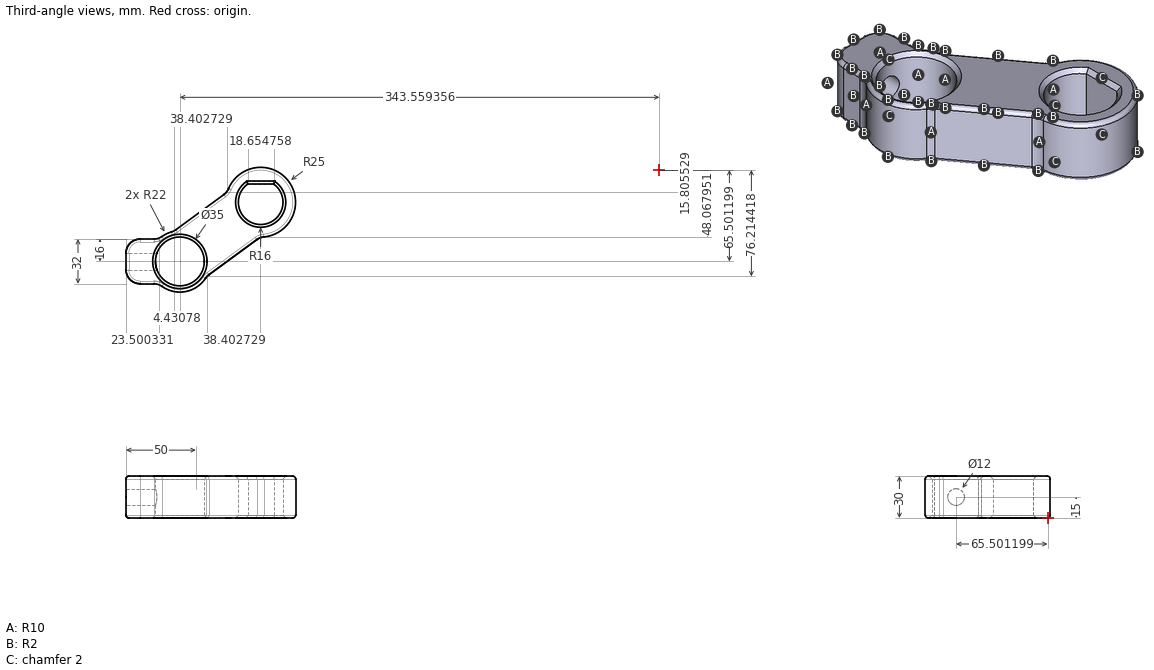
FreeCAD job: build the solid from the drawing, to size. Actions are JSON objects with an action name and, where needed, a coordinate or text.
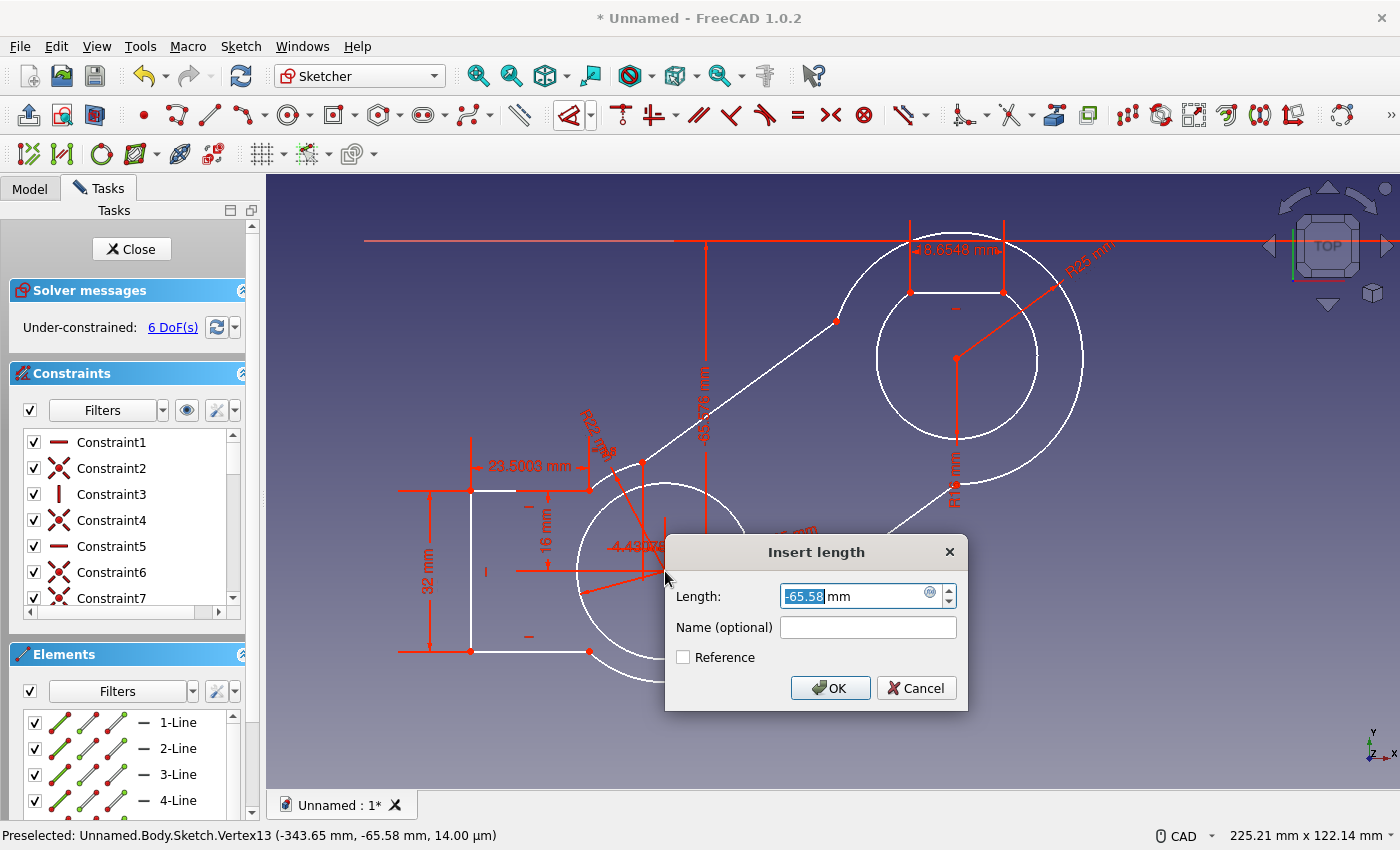
{"action": "type", "text": "-65.501199"}
{"action": "key", "text": "Return"}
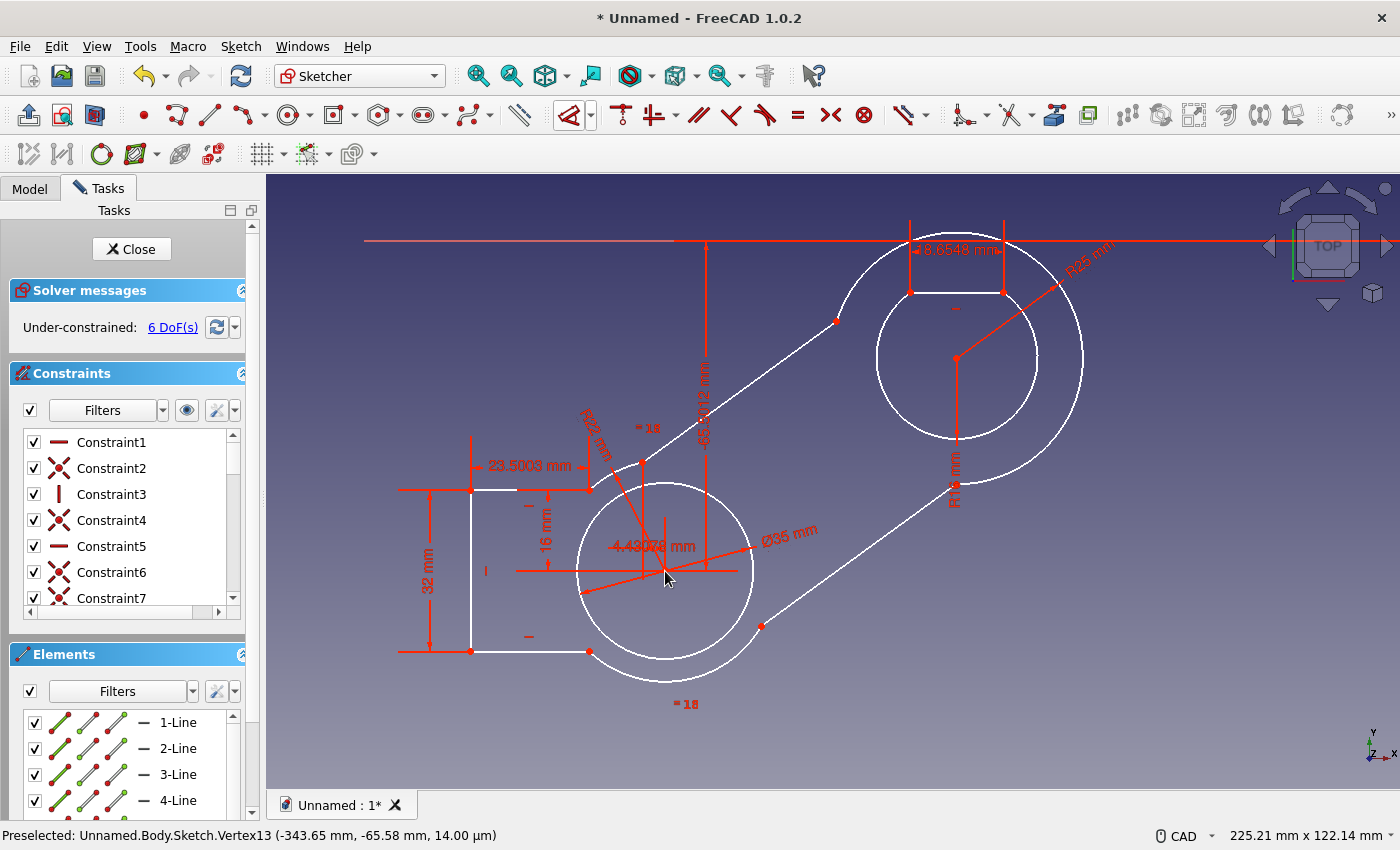
{"action": "left_click", "coordinate": [837, 321]}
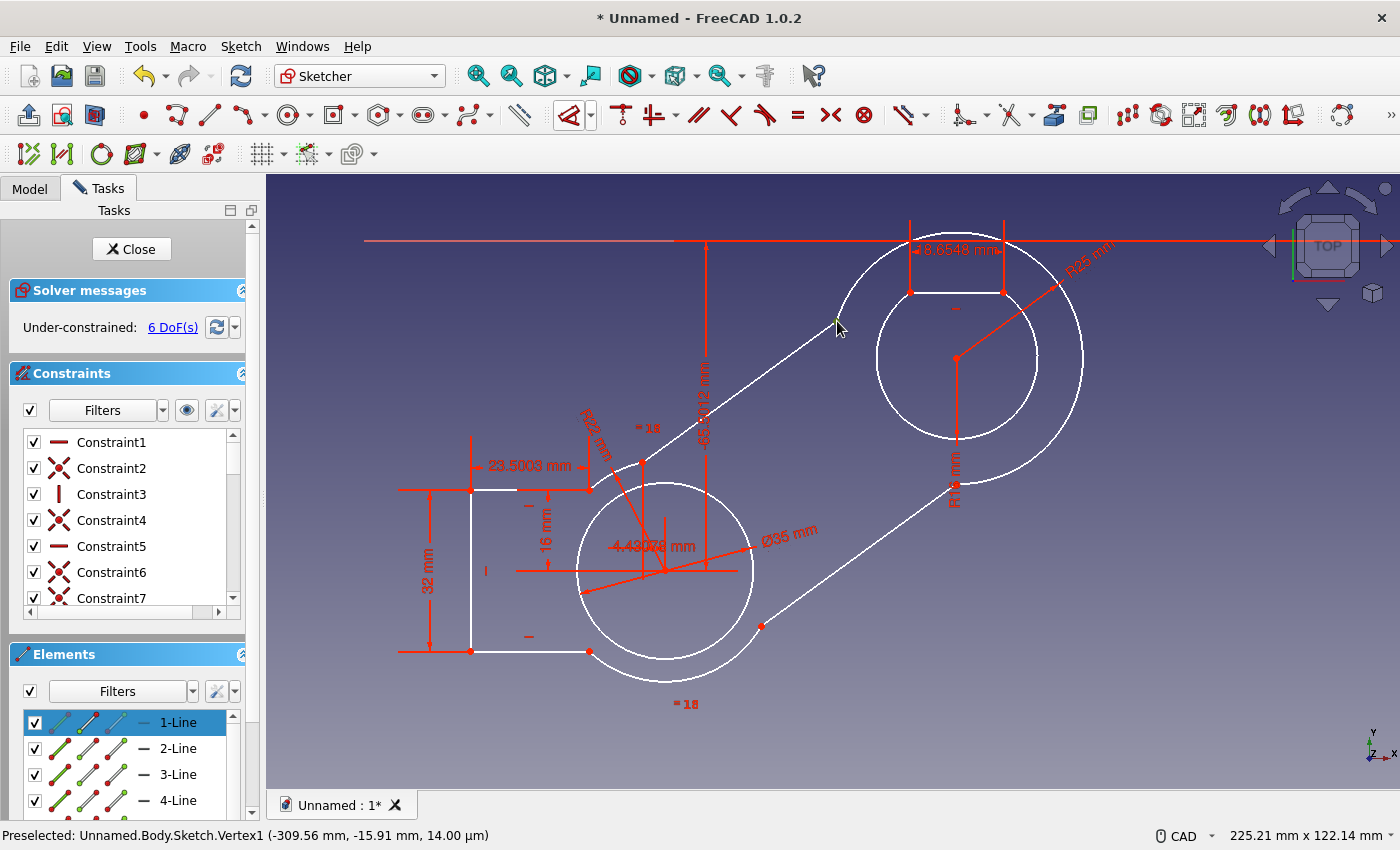
{"action": "key", "text": "i"}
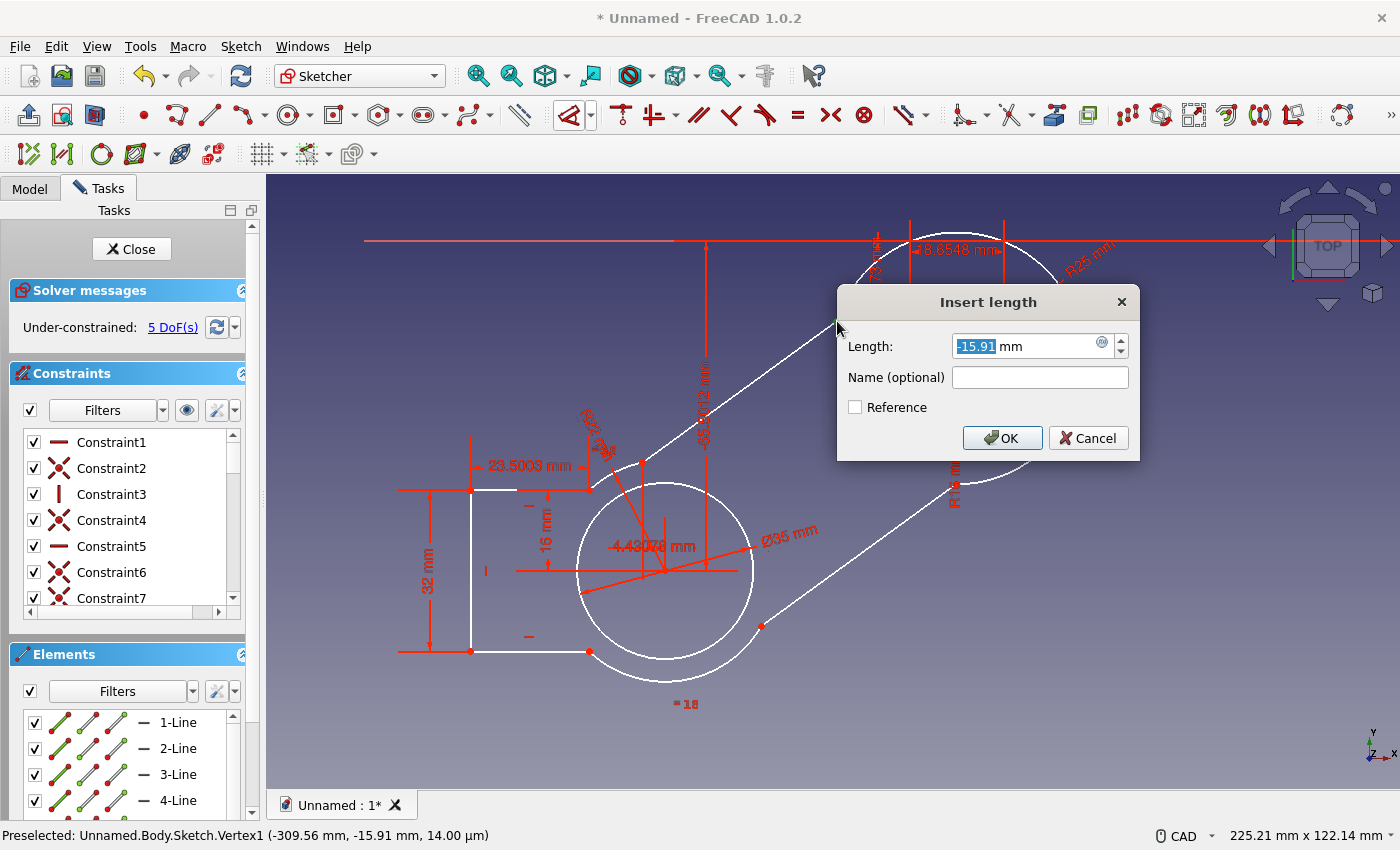
{"action": "type", "text": "-15.805529"}
{"action": "key", "text": "Return"}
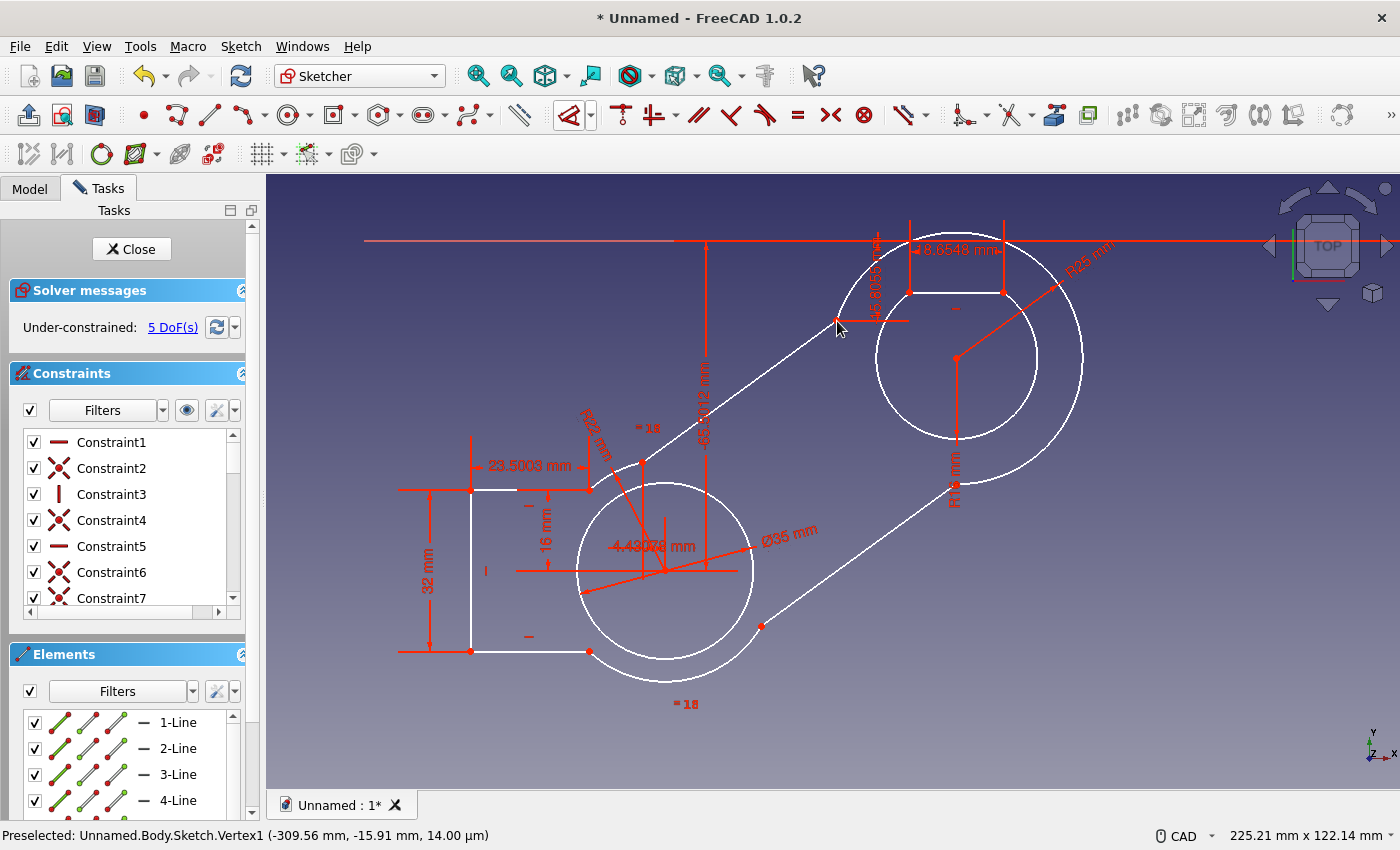
{"action": "left_click", "coordinate": [761, 626]}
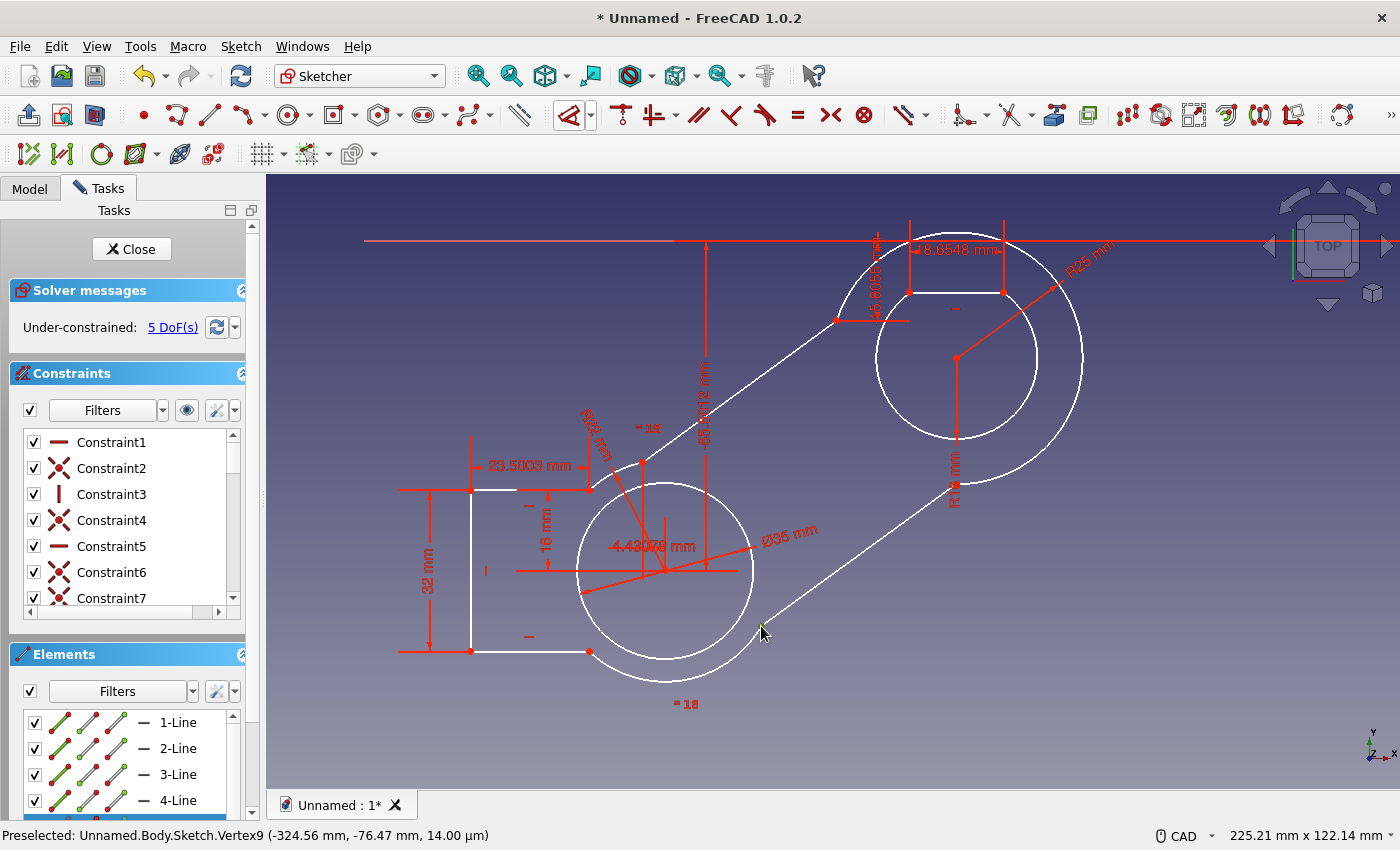
{"action": "left_click", "coordinate": [590, 116]}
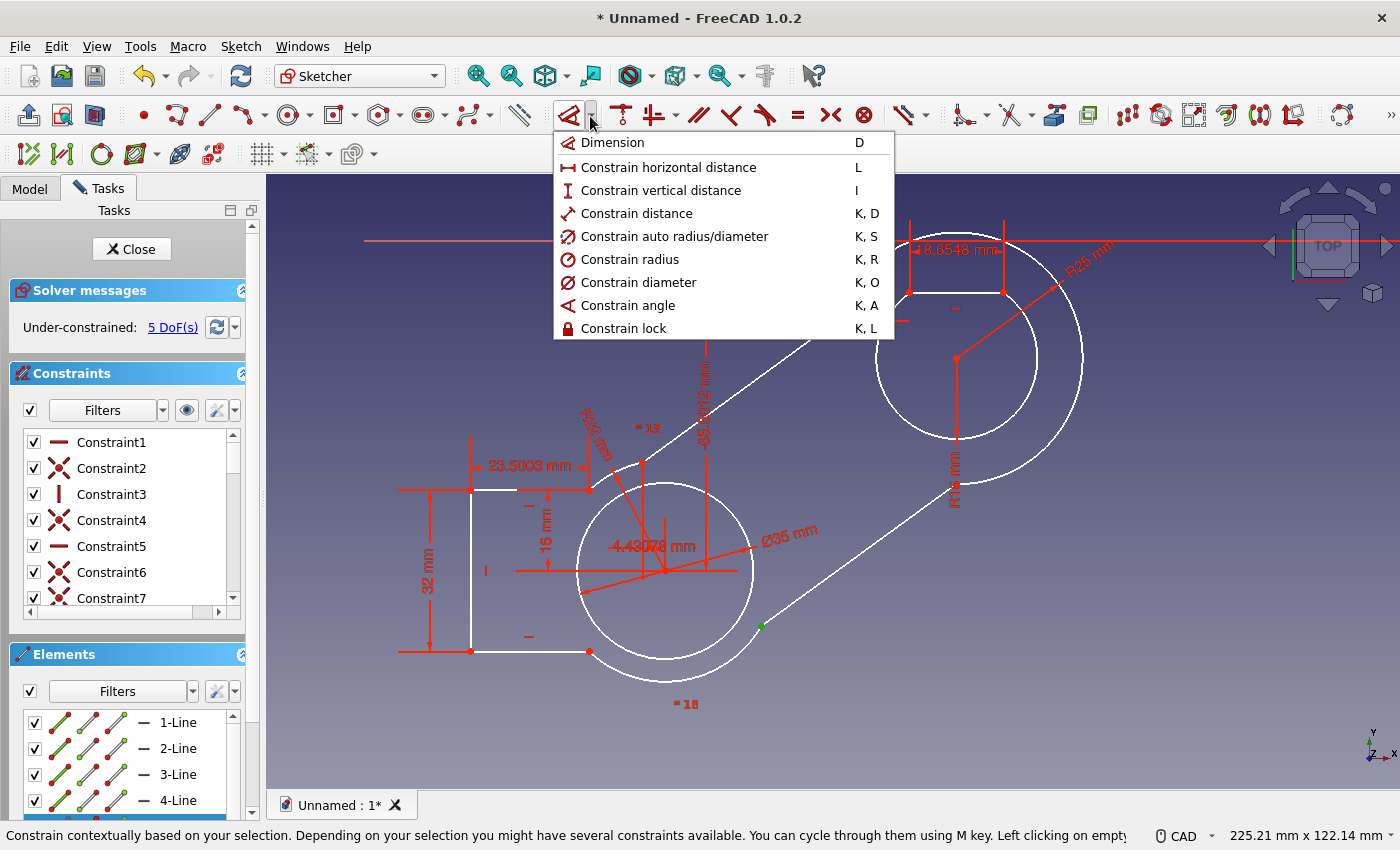
{"action": "left_click", "coordinate": [724, 190]}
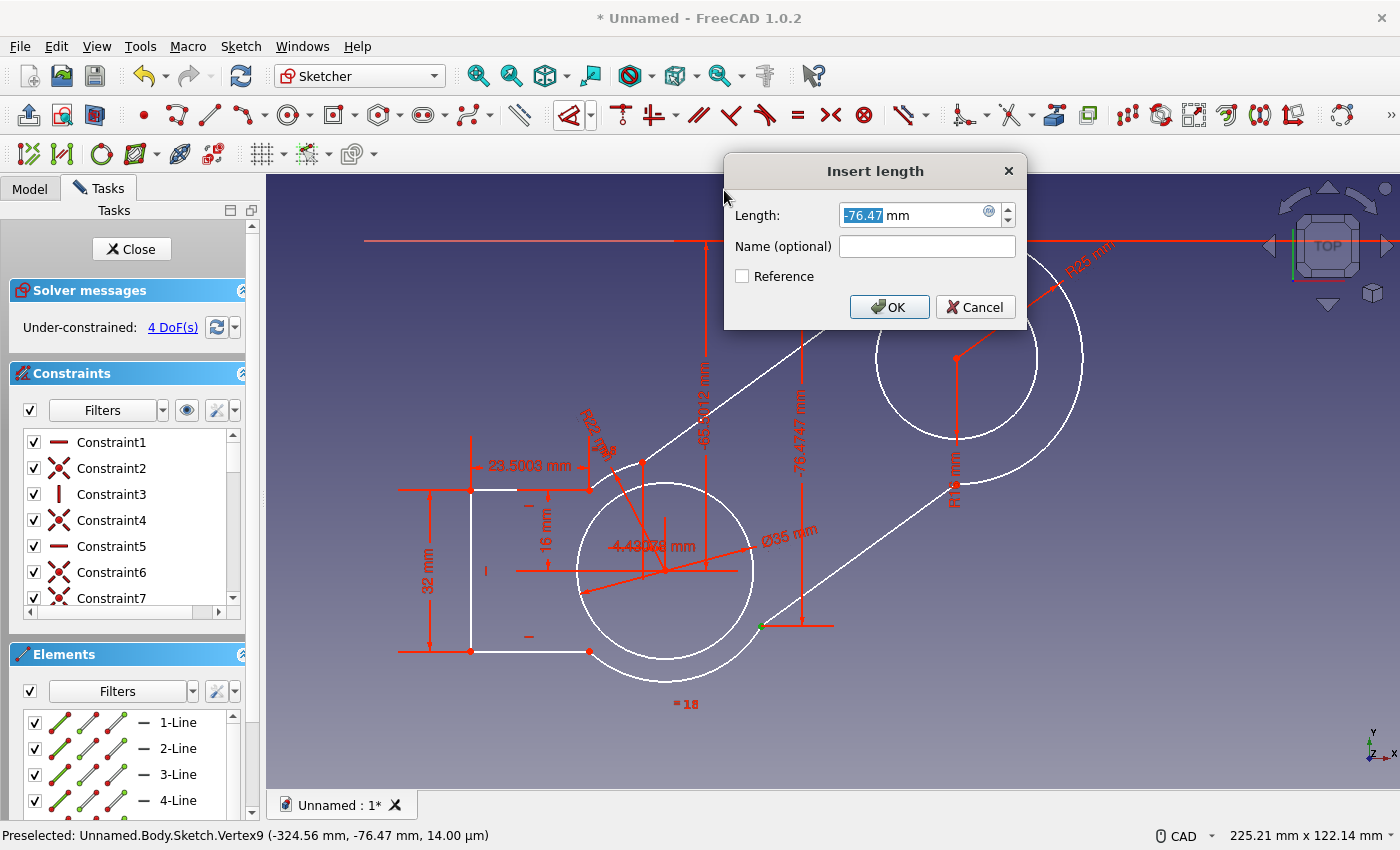
{"action": "type", "text": "-76.214418"}
{"action": "key", "text": "Return"}